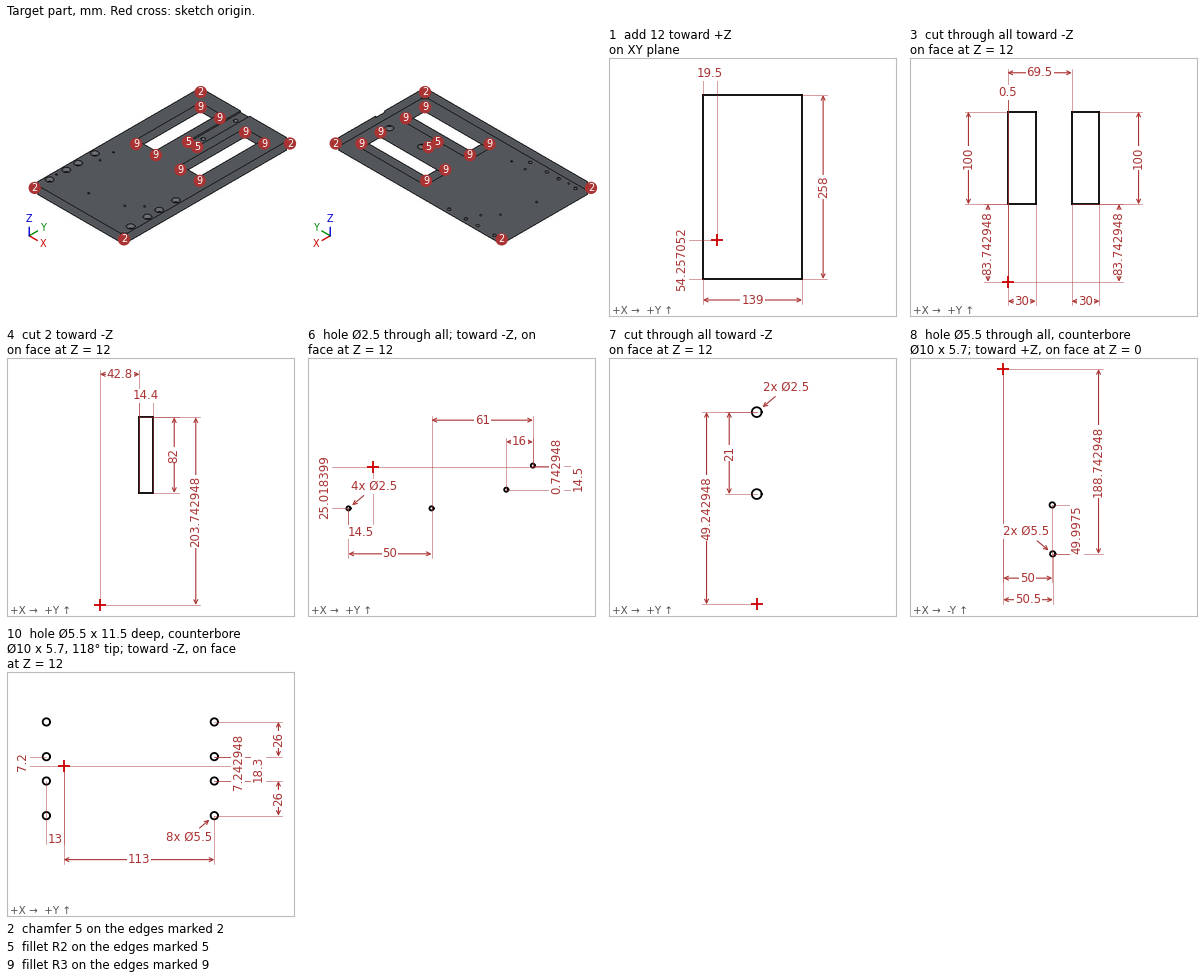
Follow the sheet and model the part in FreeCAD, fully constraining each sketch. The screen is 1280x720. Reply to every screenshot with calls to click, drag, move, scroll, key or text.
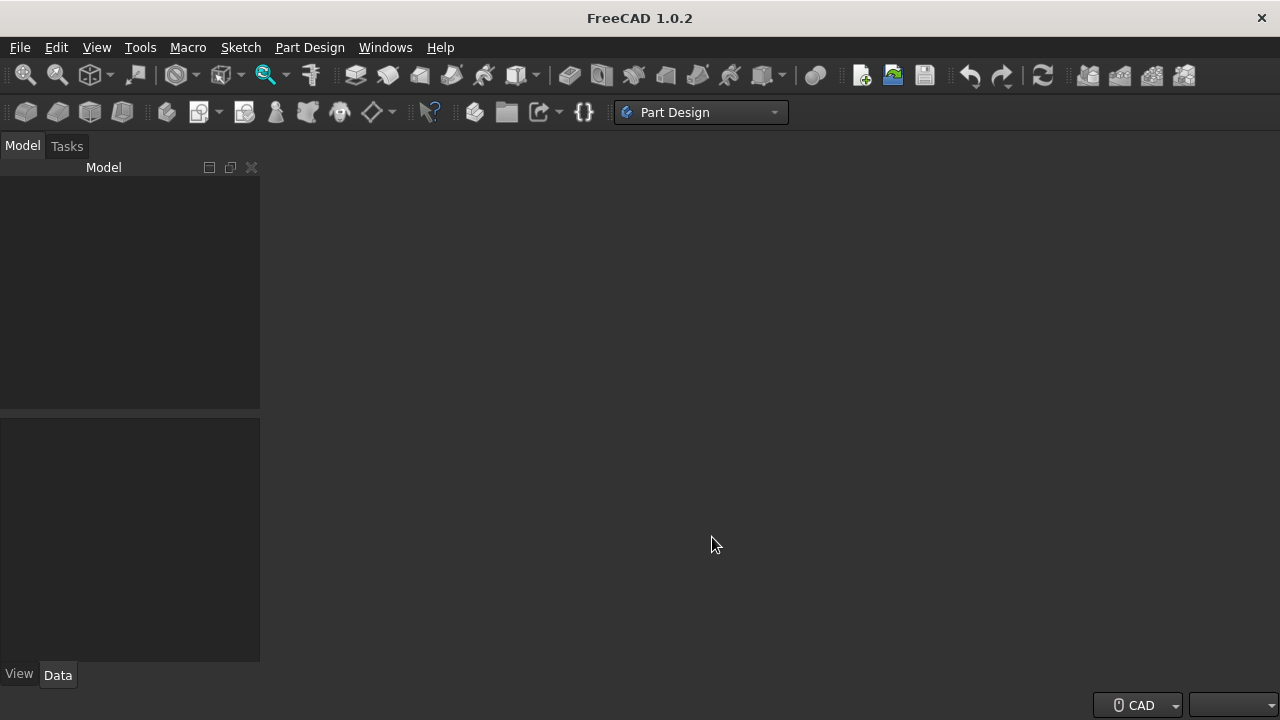
key(ctrl+n)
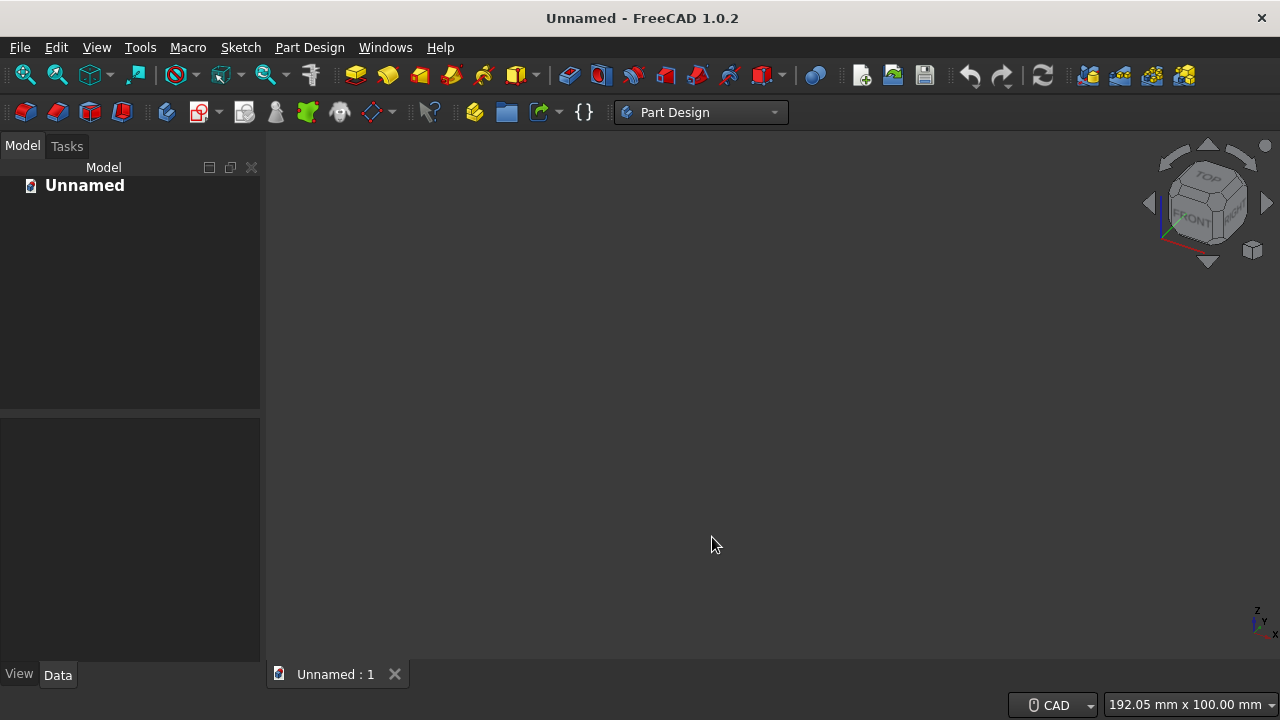
click(200, 112)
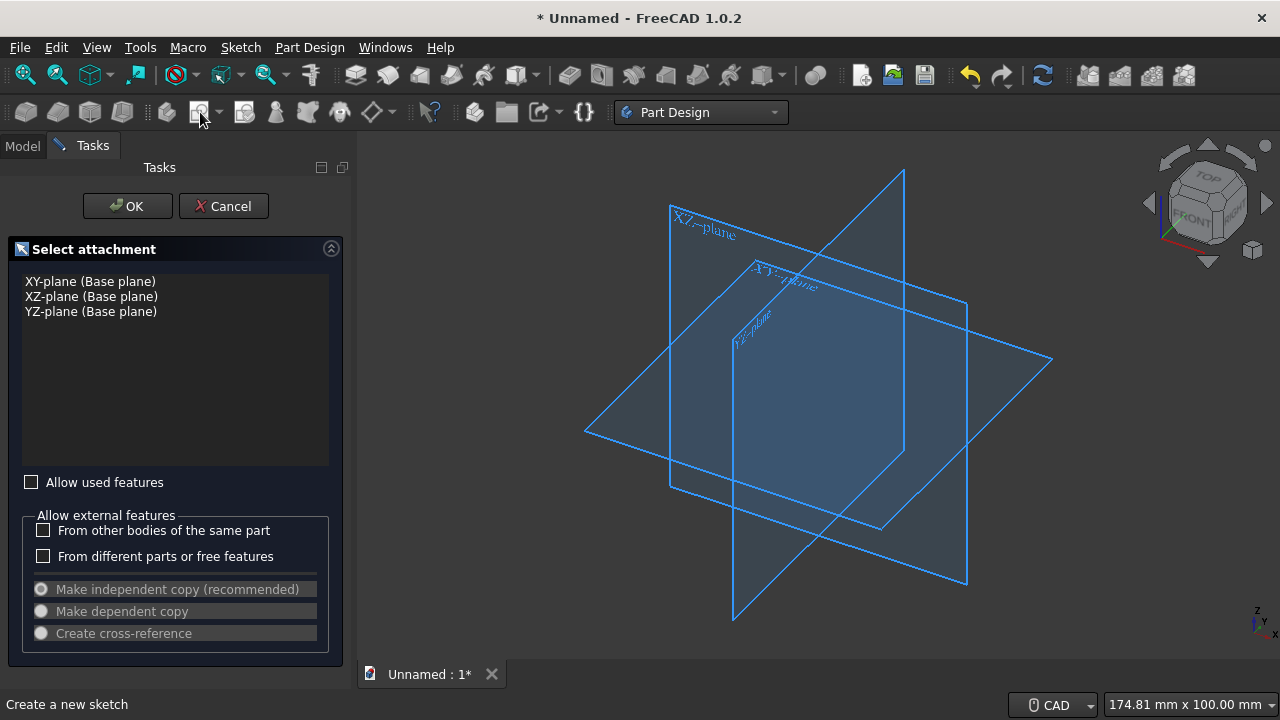
click(82, 282)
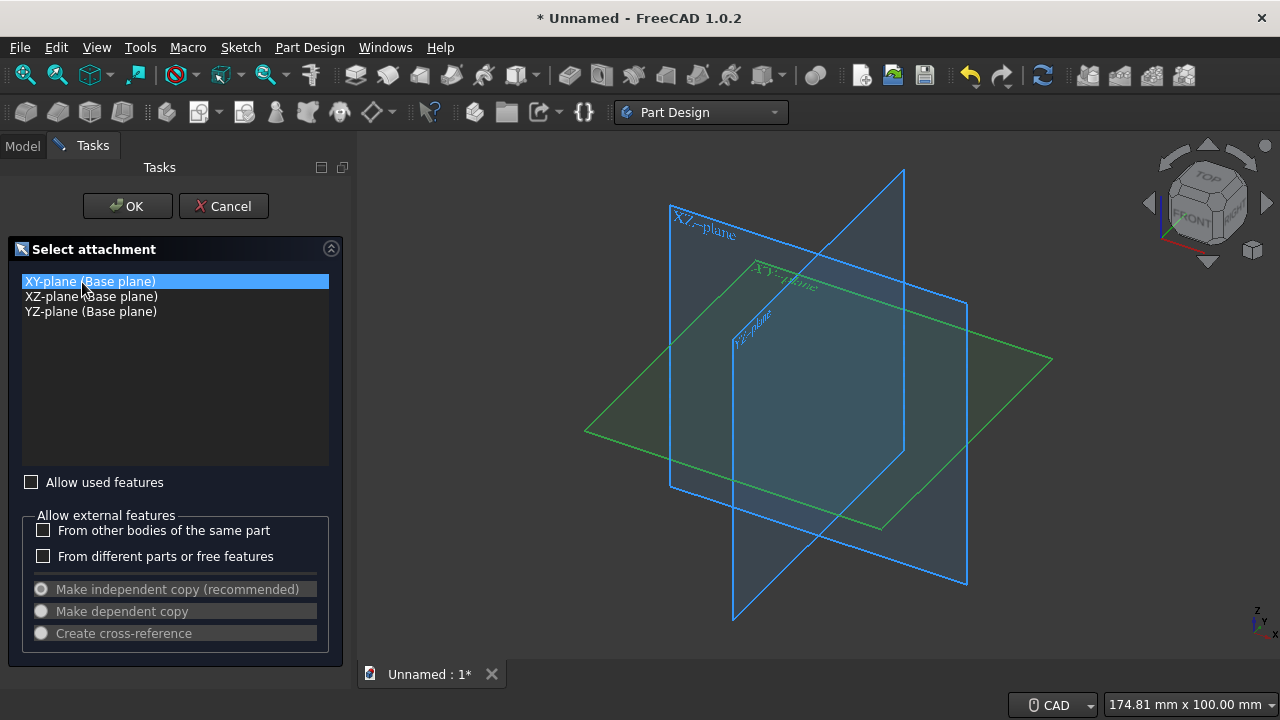
click(128, 206)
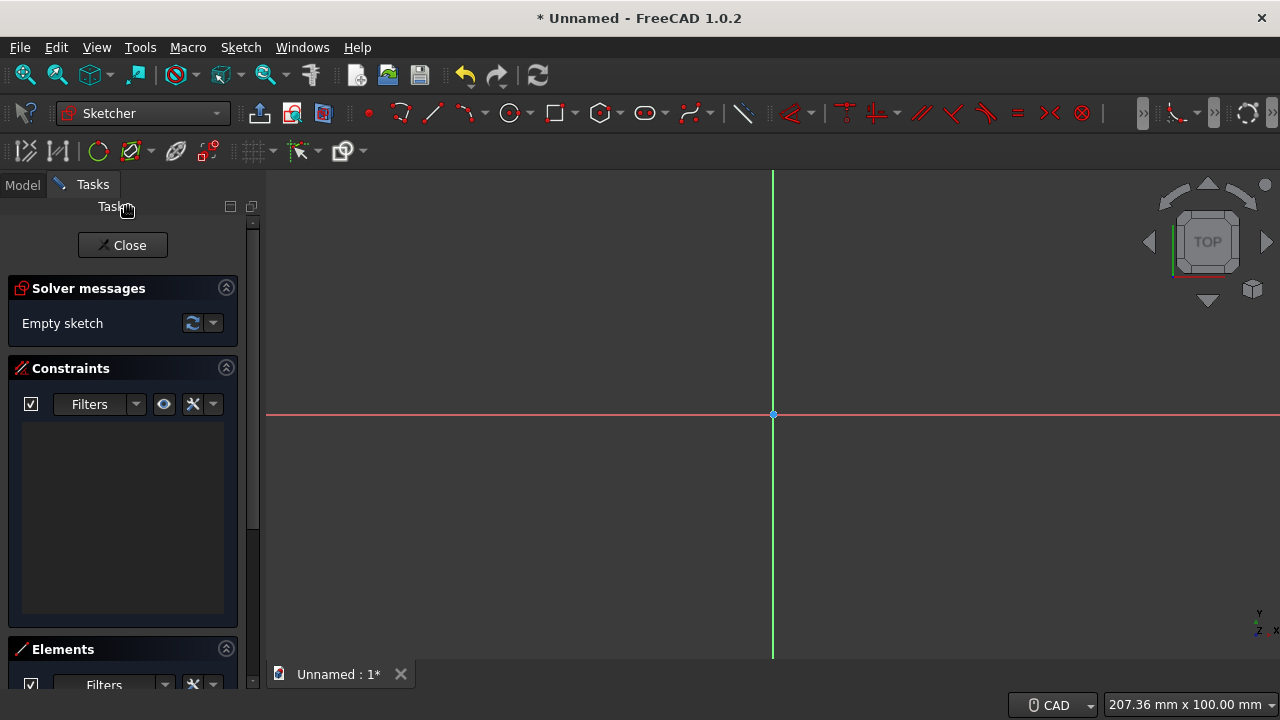
scroll(602, 534, down, 7)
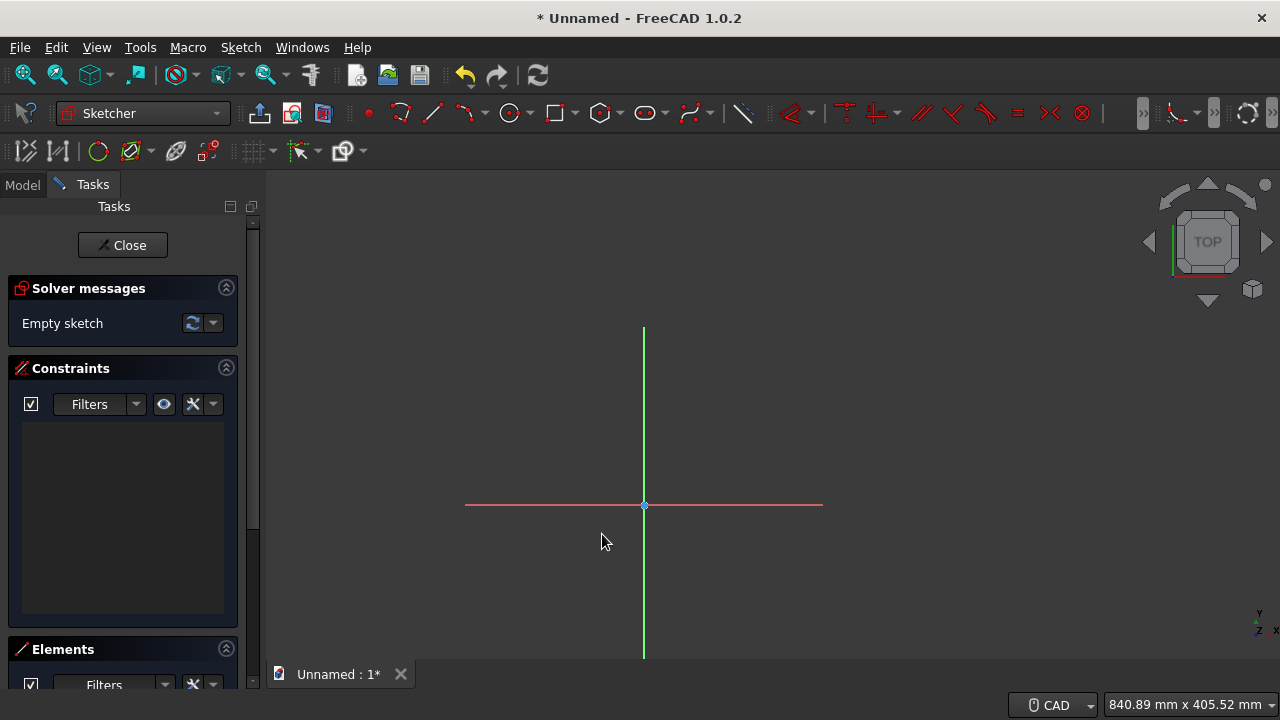
key(g)
key(r)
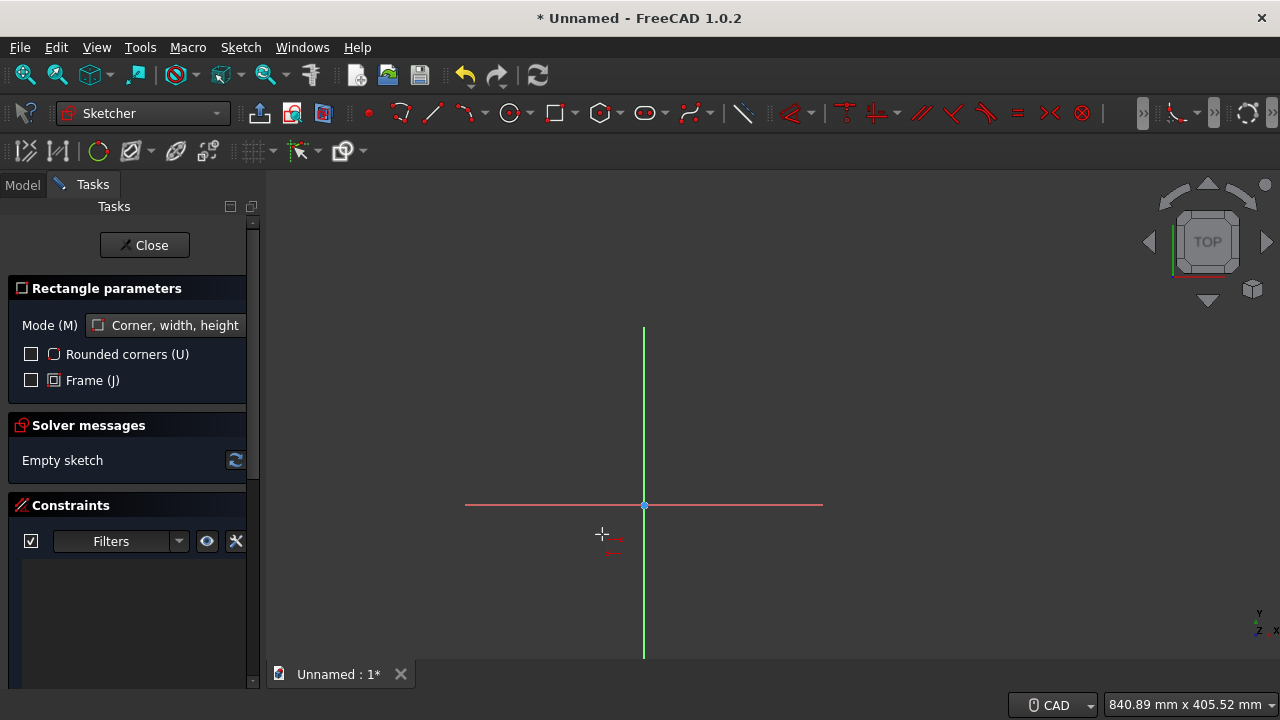
click(621, 259)
move(789, 571)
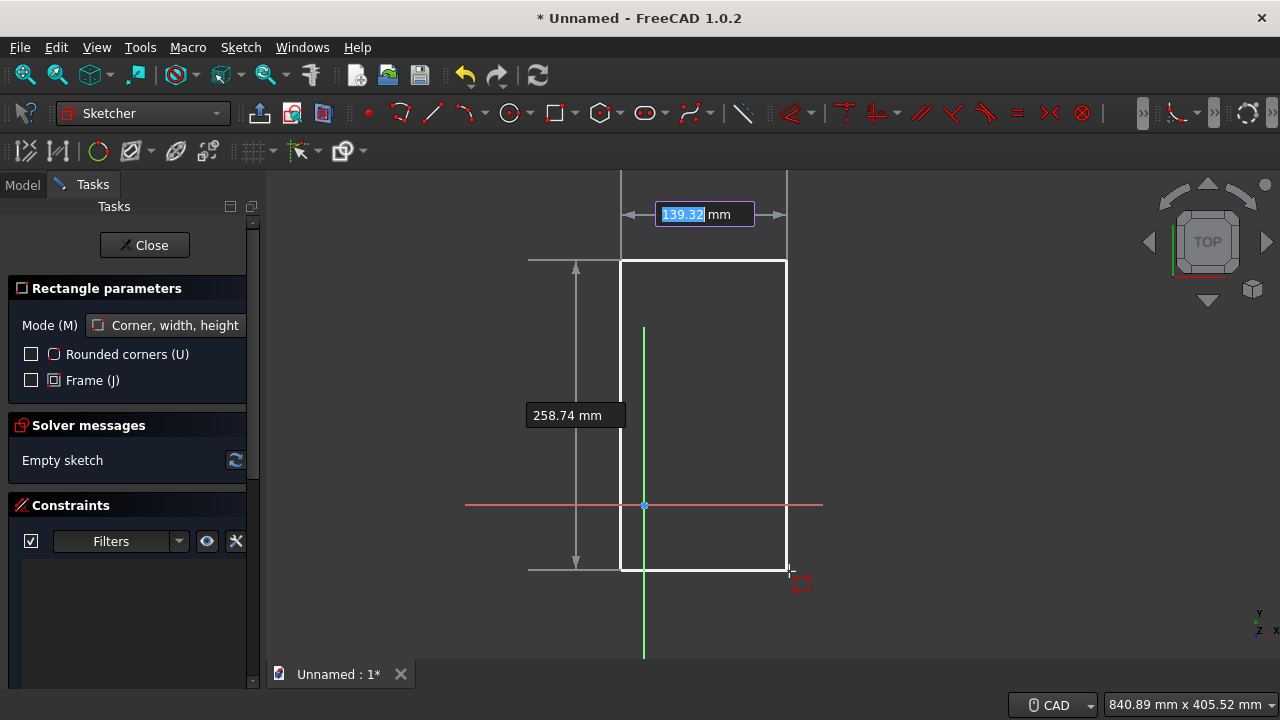
text(139)
key(Tab)
text(258)
key(Return)
key(Escape)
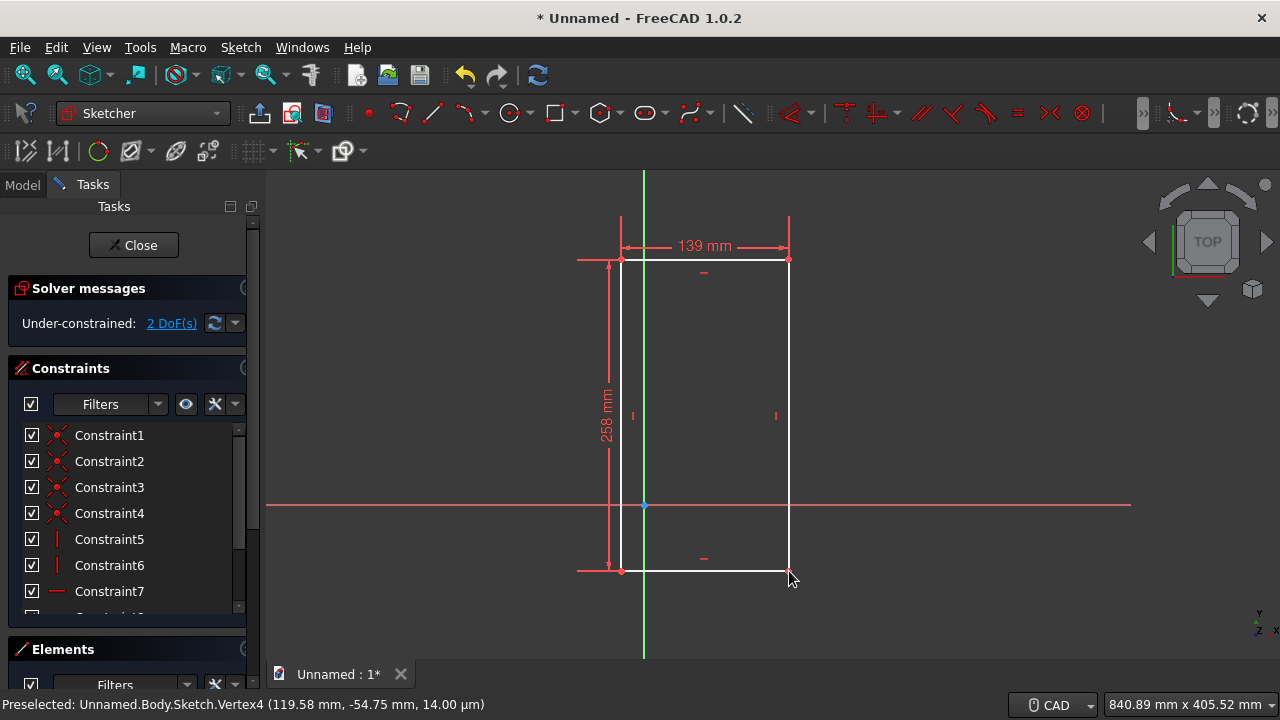
key(d)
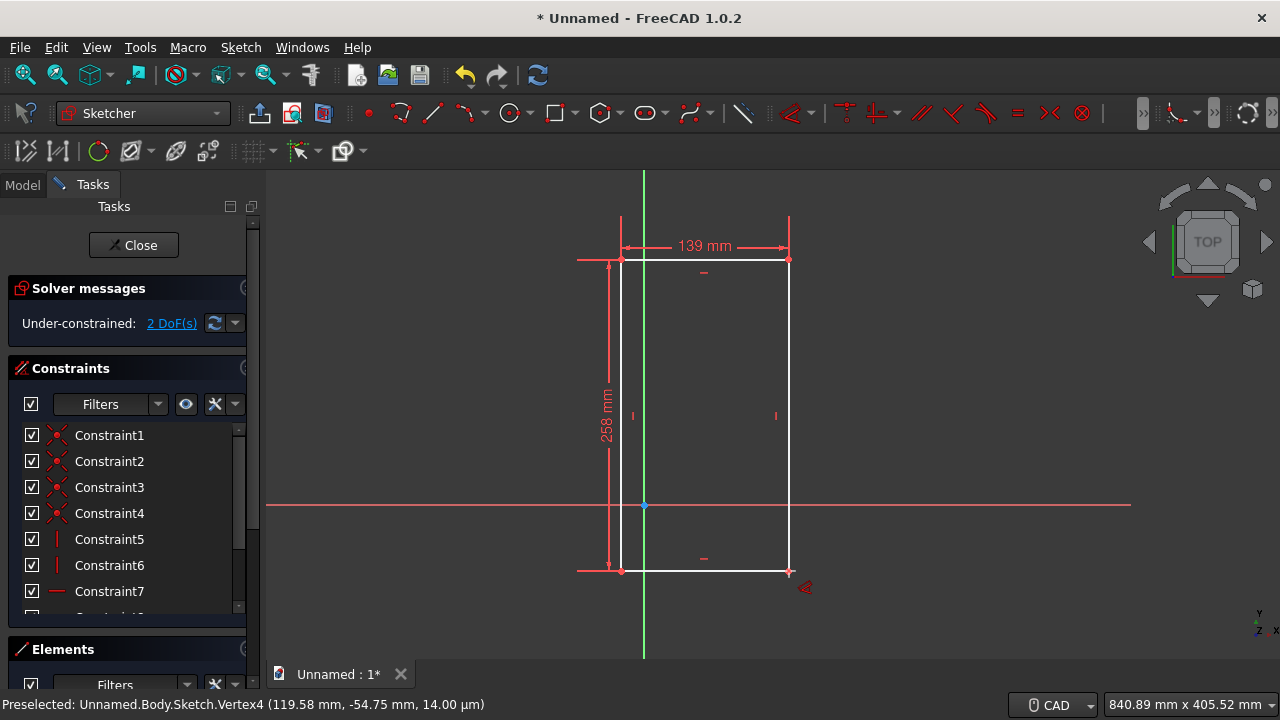
scroll(621, 260, up, 3)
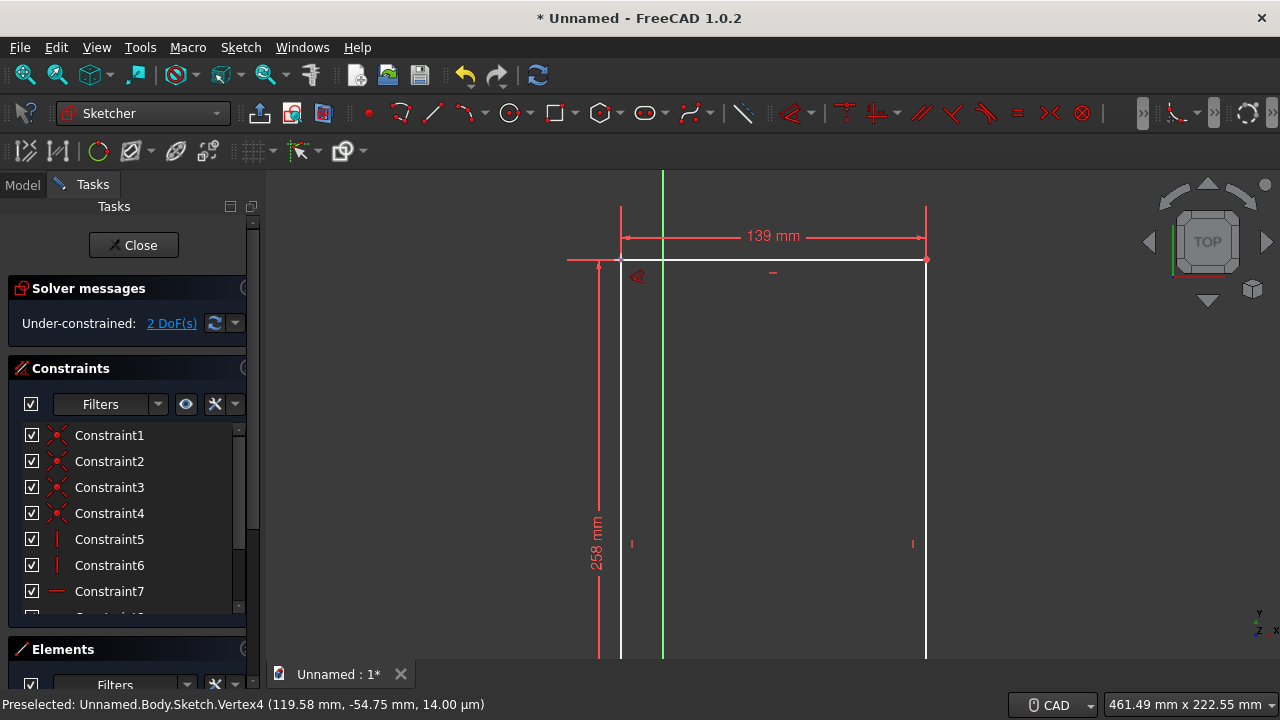
click(621, 260)
click(642, 226)